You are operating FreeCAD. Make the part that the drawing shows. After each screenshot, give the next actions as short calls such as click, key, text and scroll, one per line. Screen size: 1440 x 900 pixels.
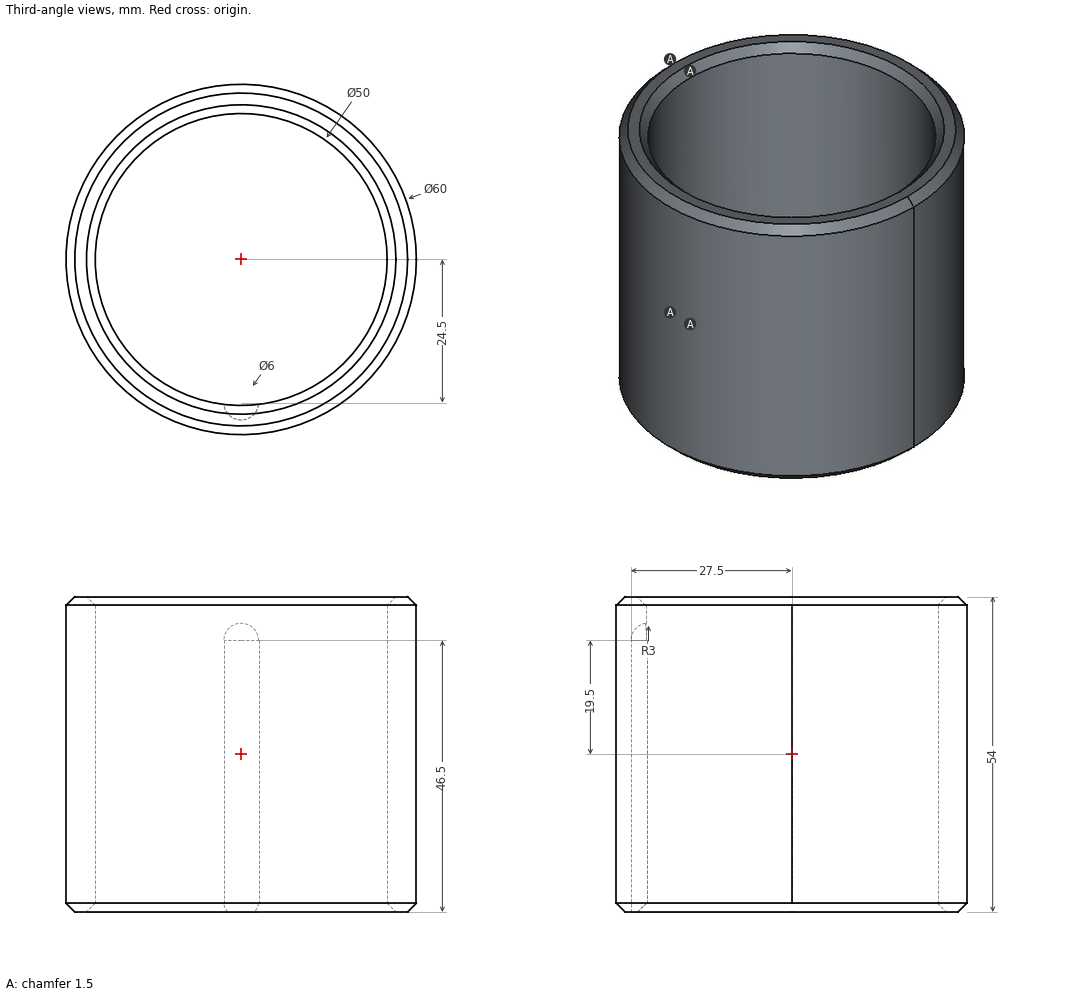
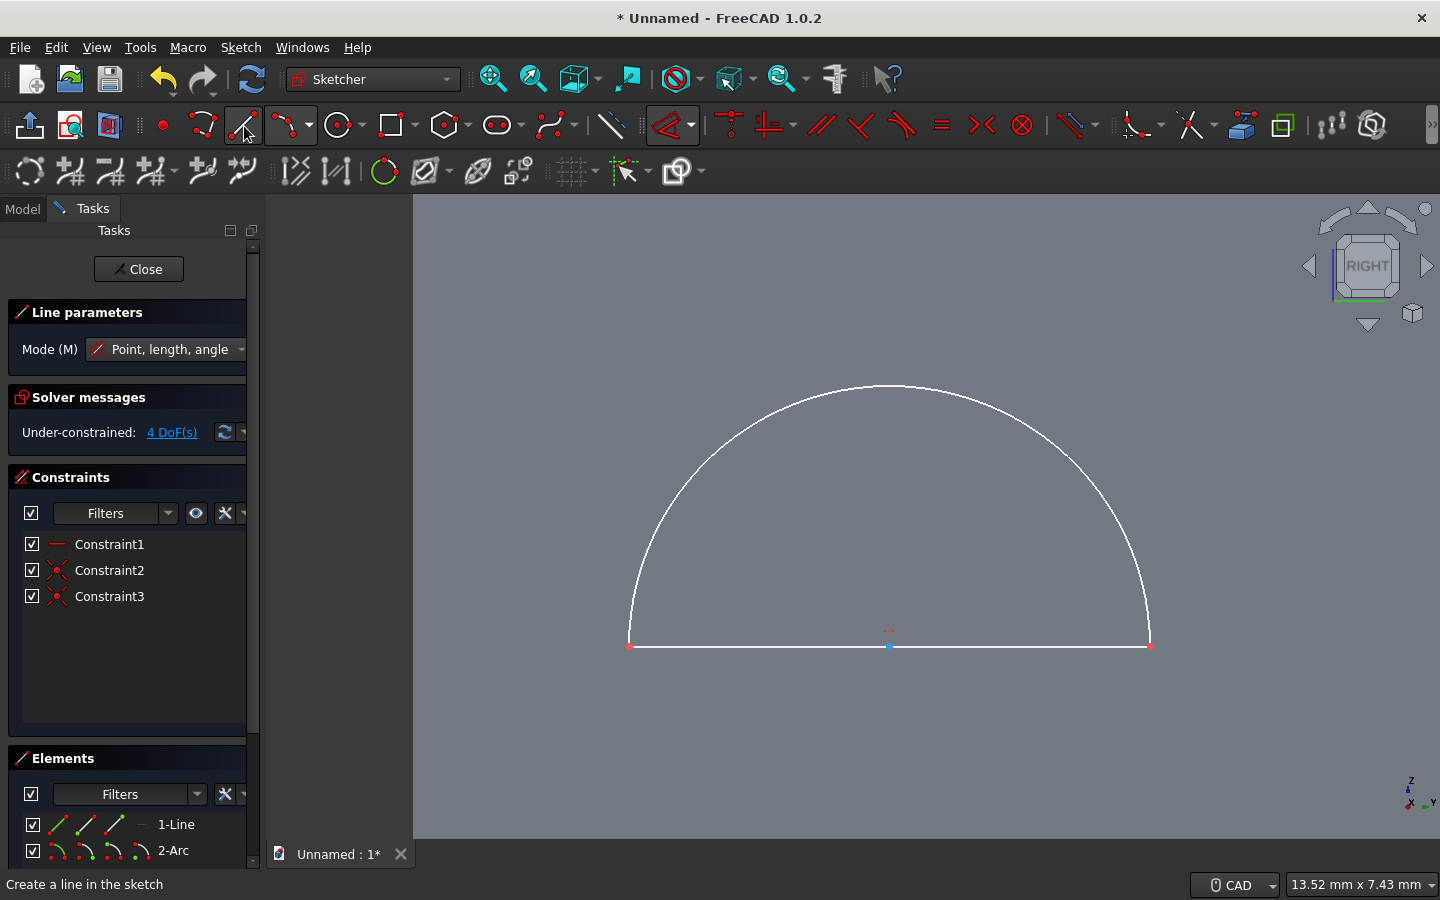
click(577, 646)
click(421, 646)
key(Escape)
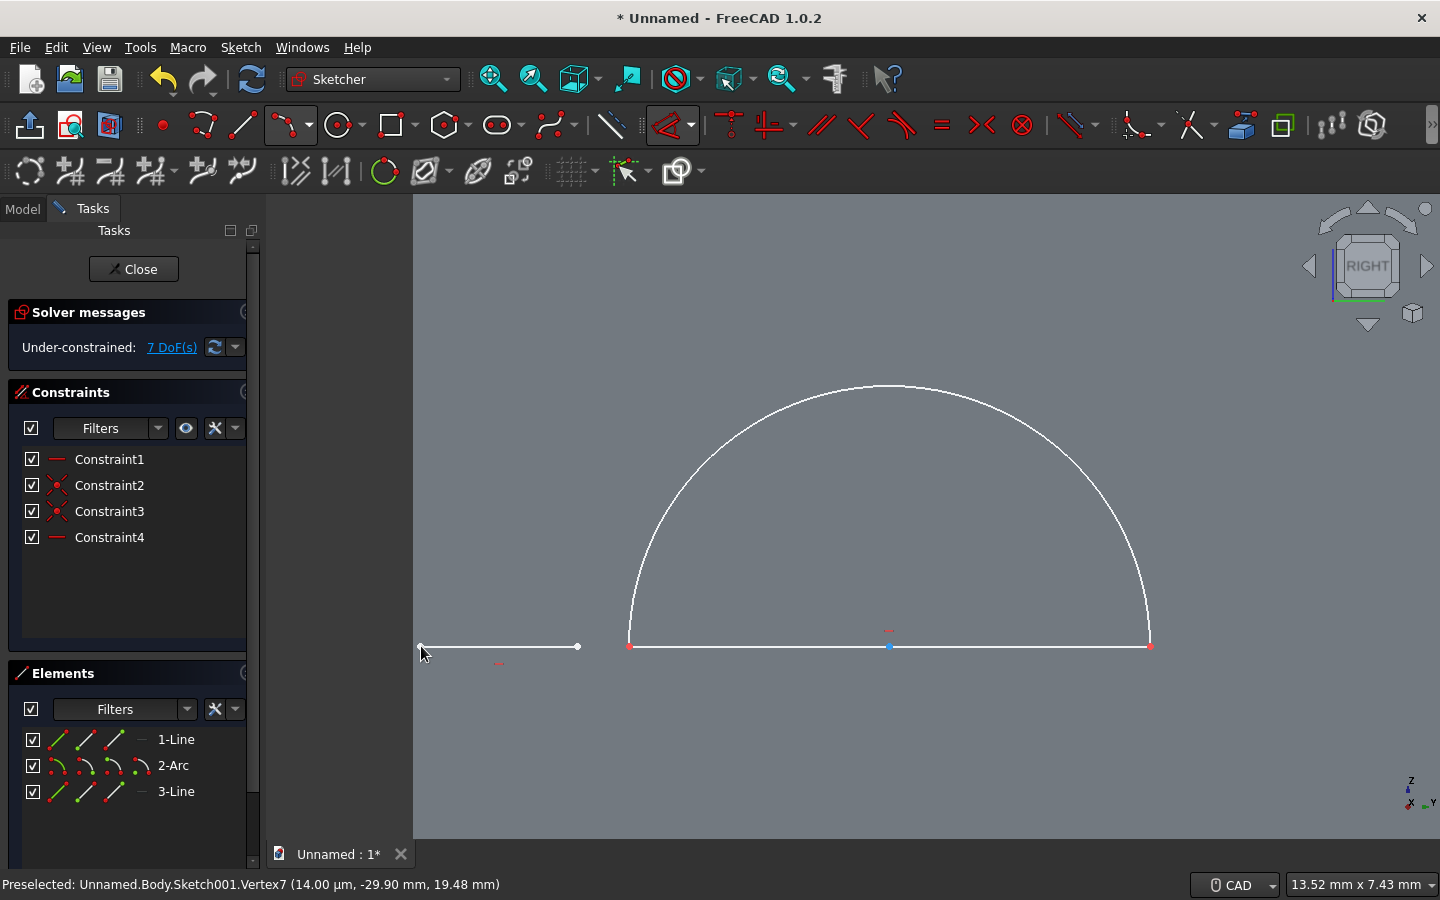
click(530, 647)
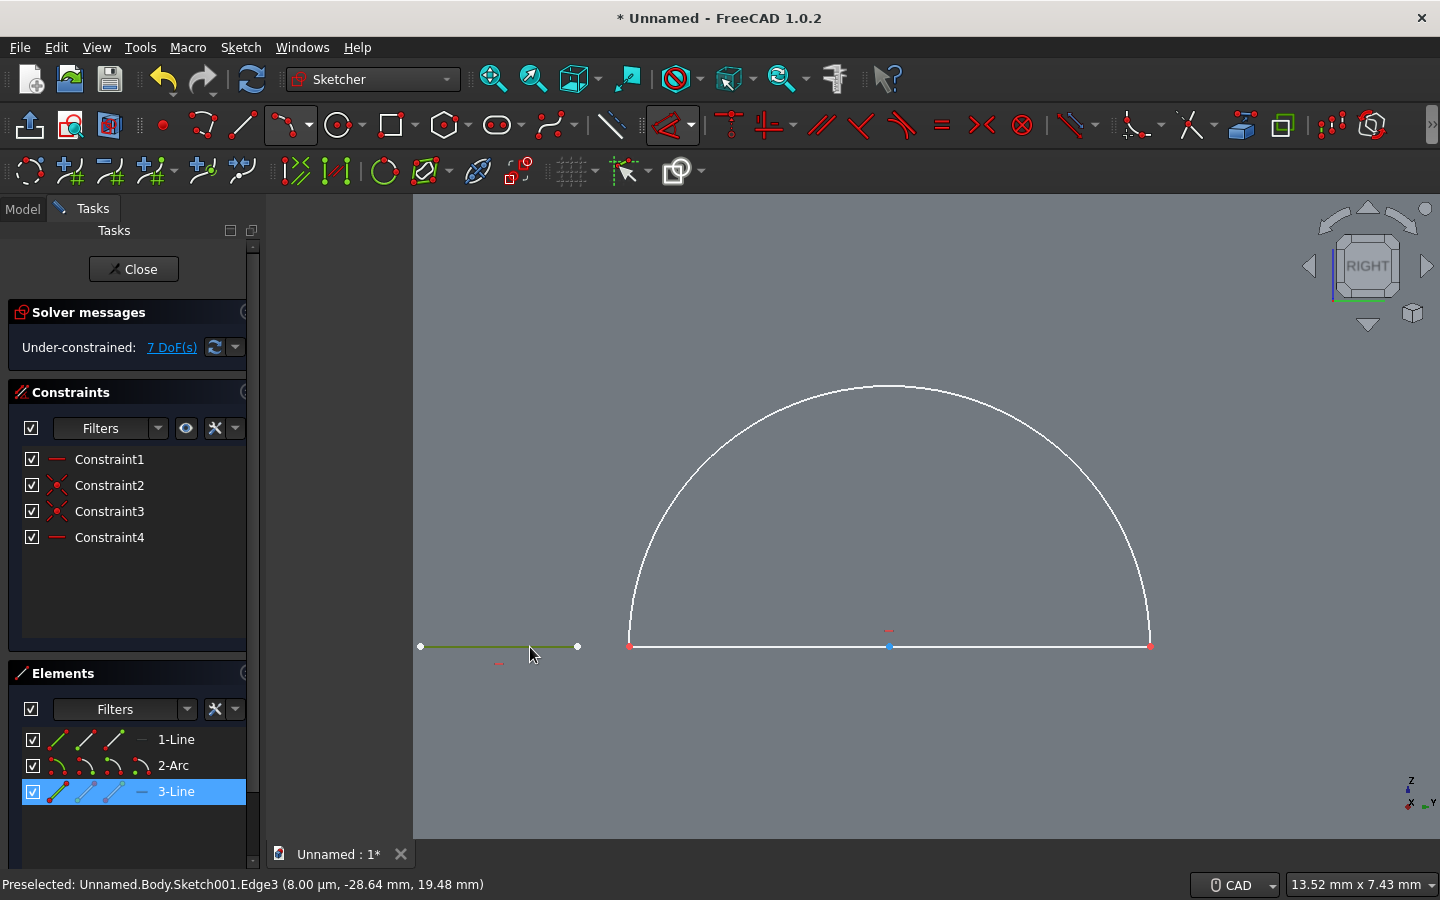
key(g)
key(n)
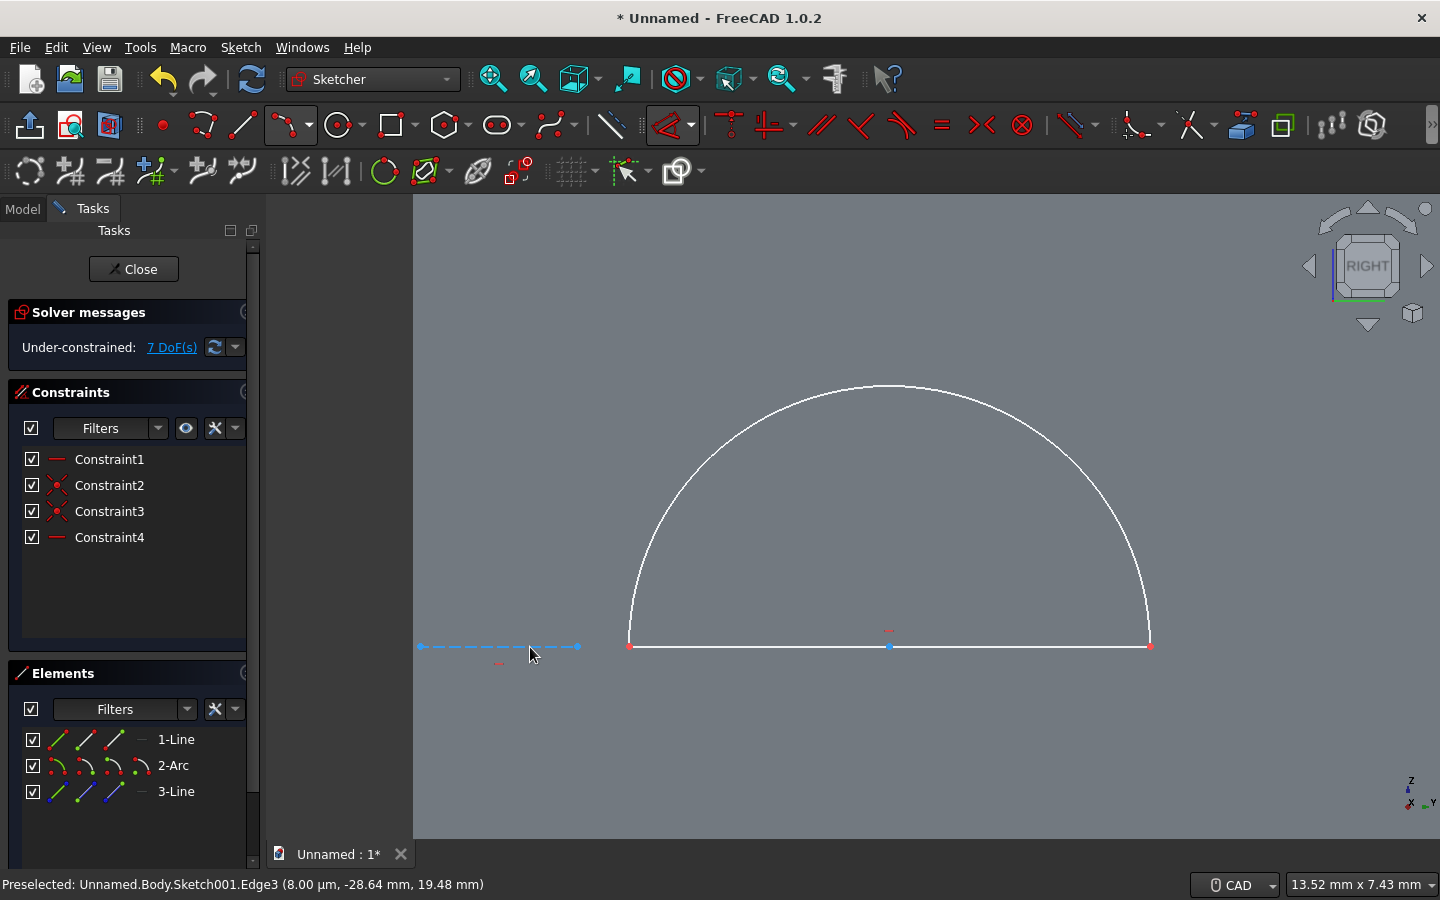
click(1043, 436)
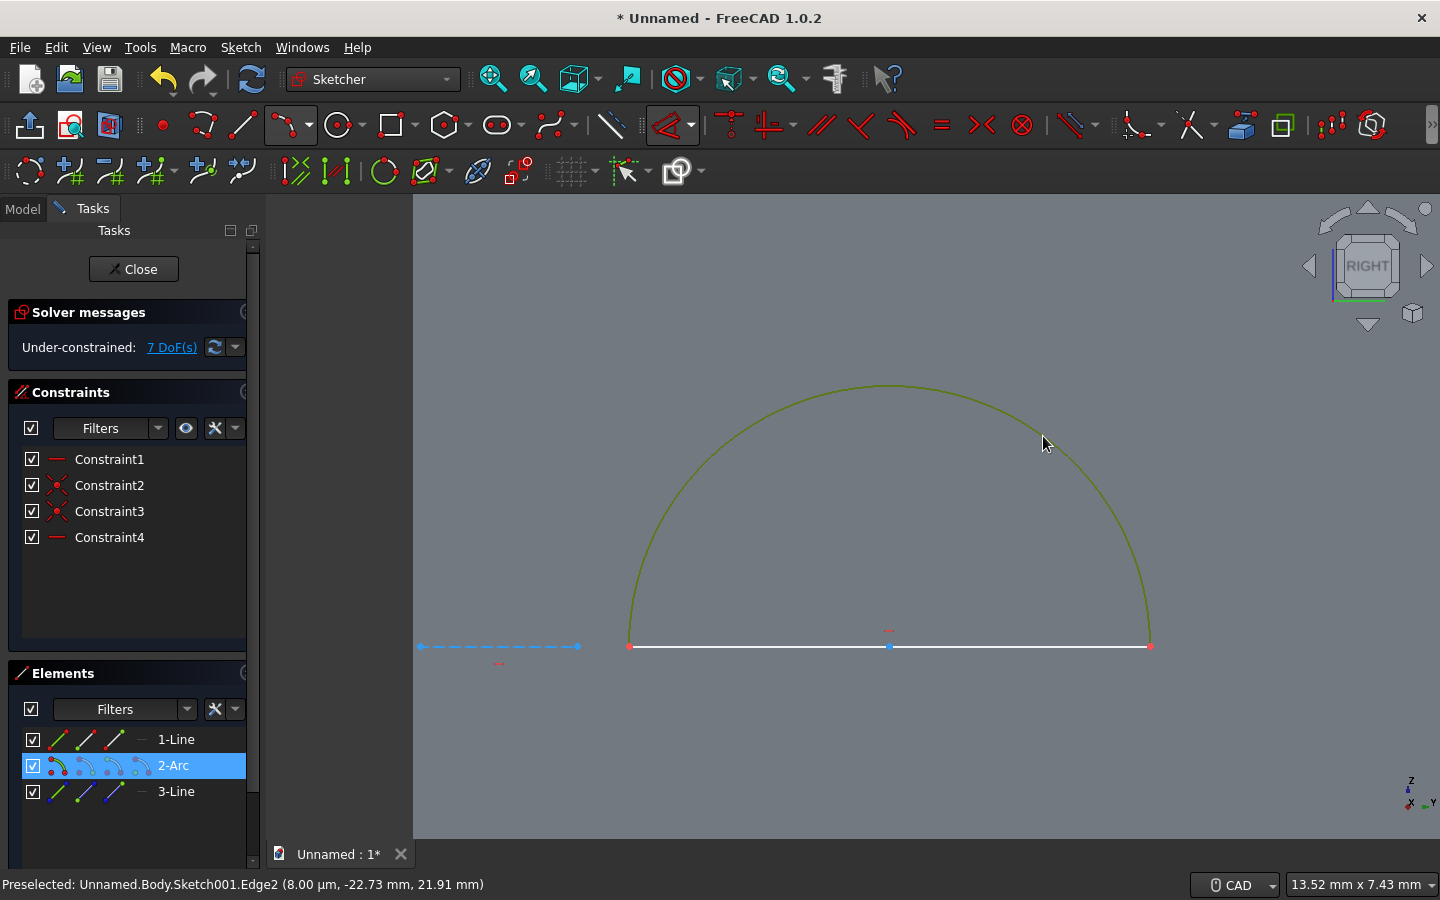
key(k)
key(r)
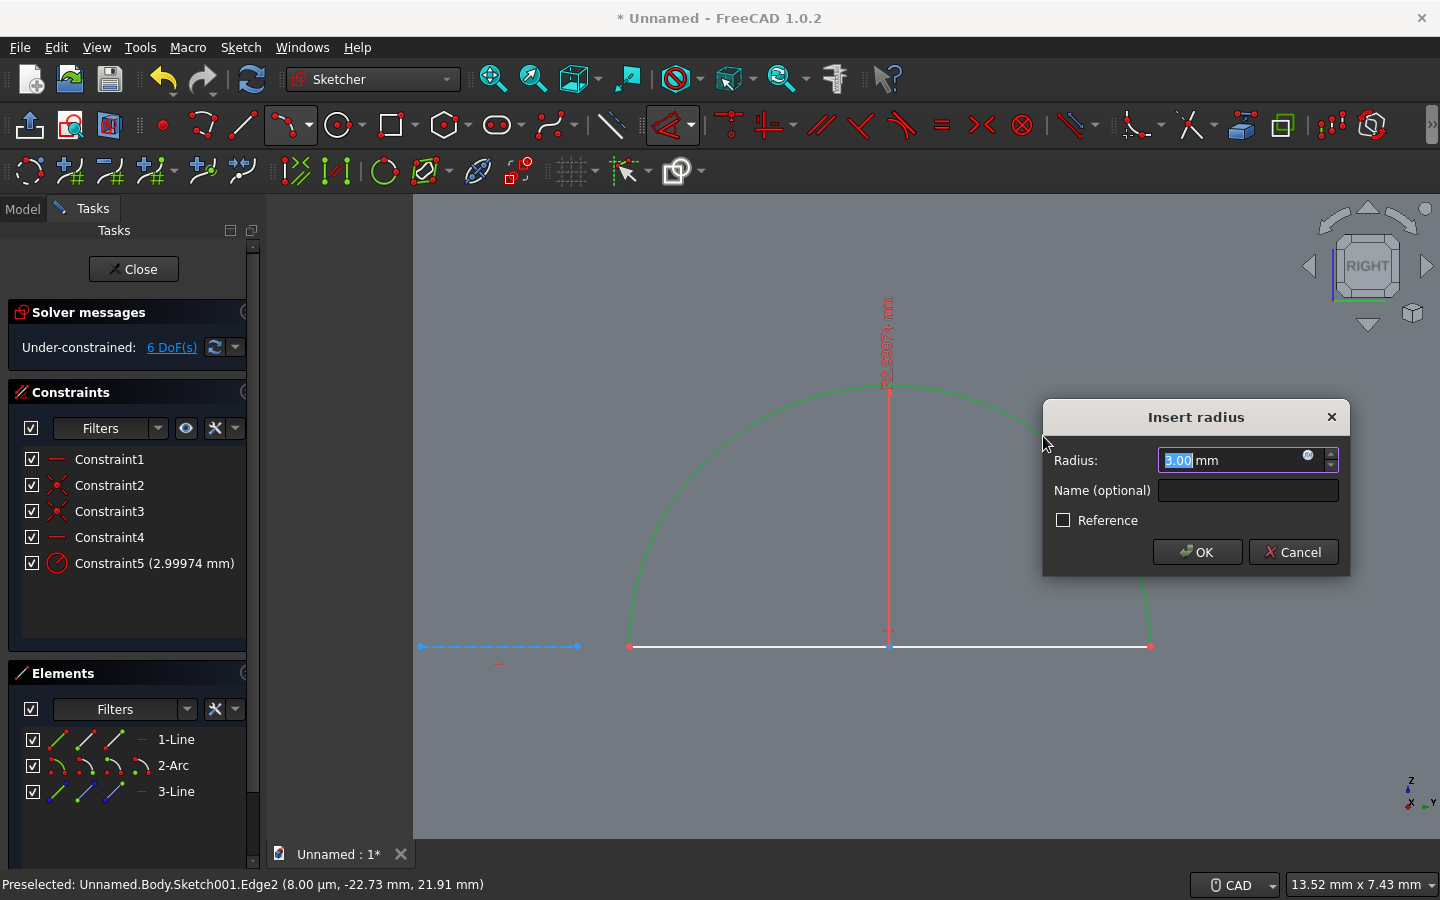
text(3)
key(Return)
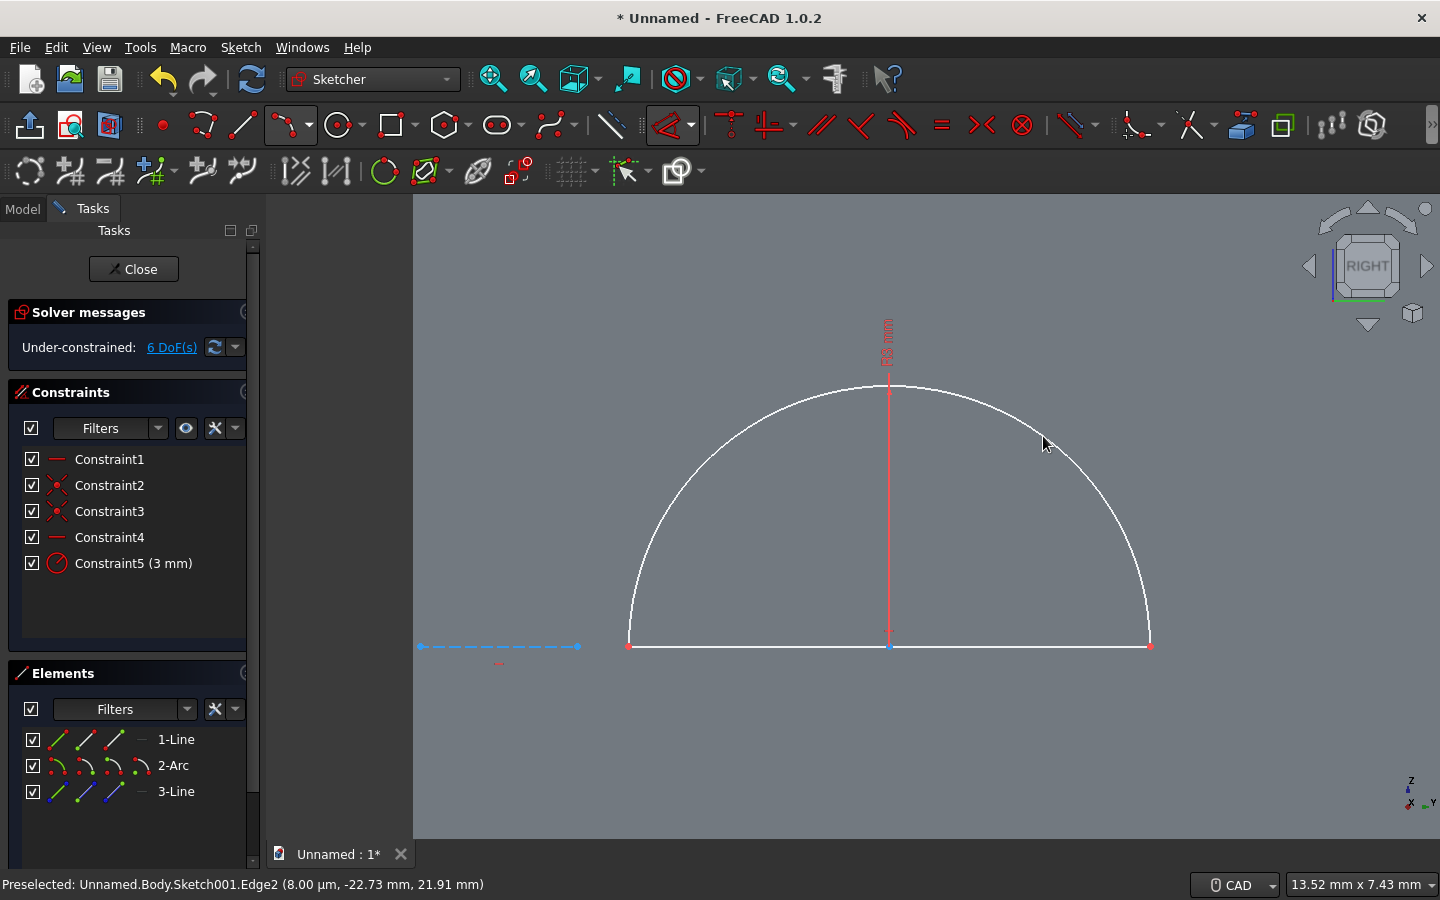
click(629, 647)